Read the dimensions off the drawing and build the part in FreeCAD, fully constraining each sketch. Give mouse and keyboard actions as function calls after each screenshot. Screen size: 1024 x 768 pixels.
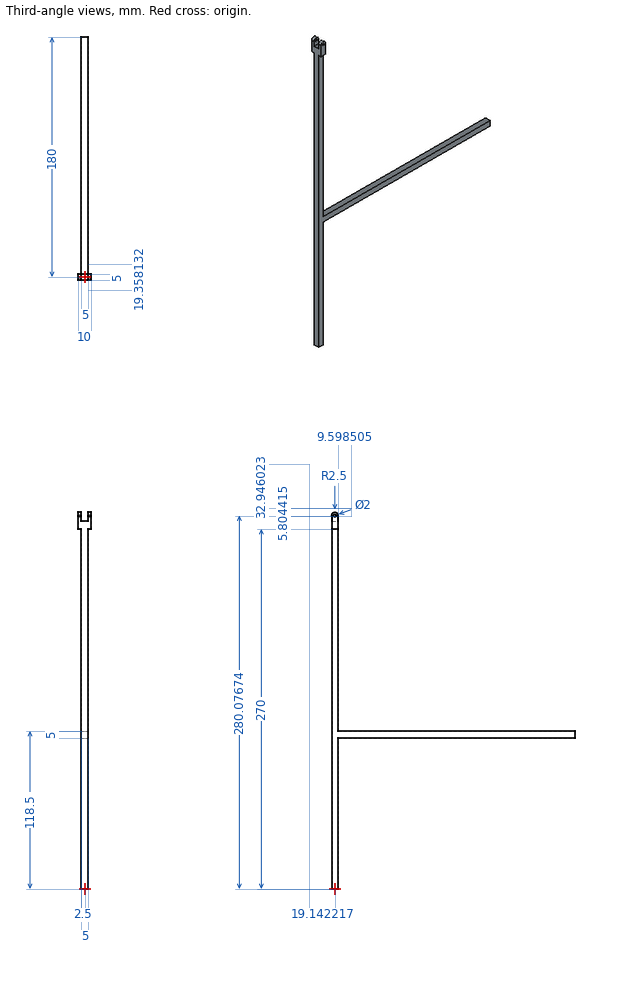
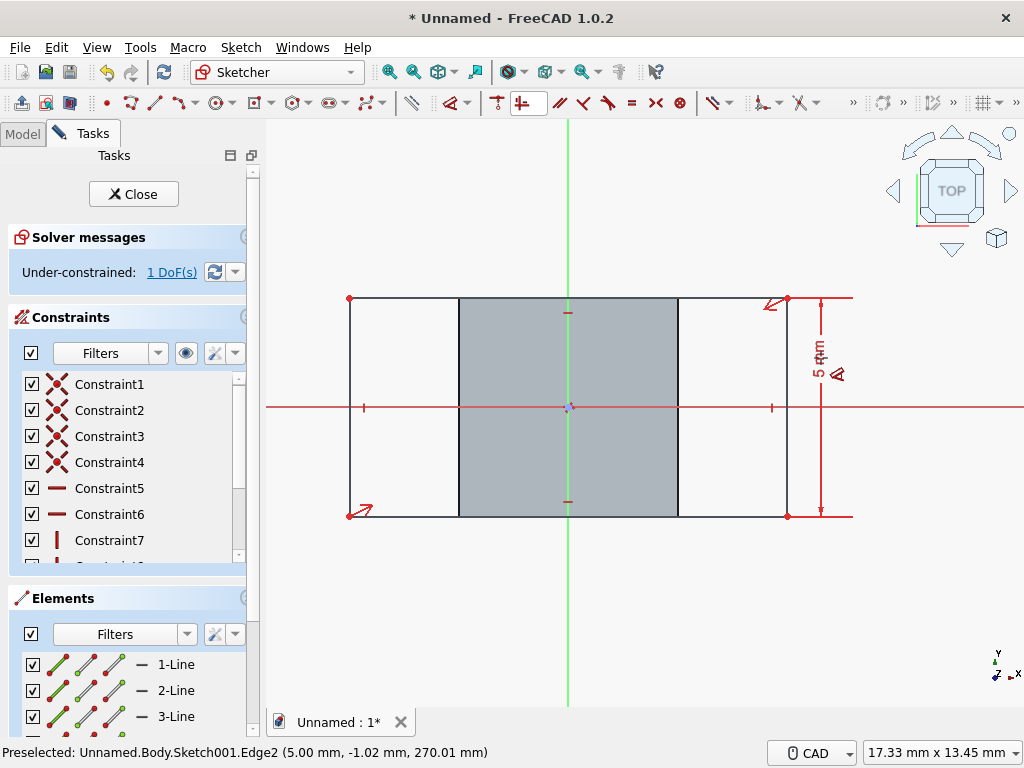
click(481, 517)
click(468, 551)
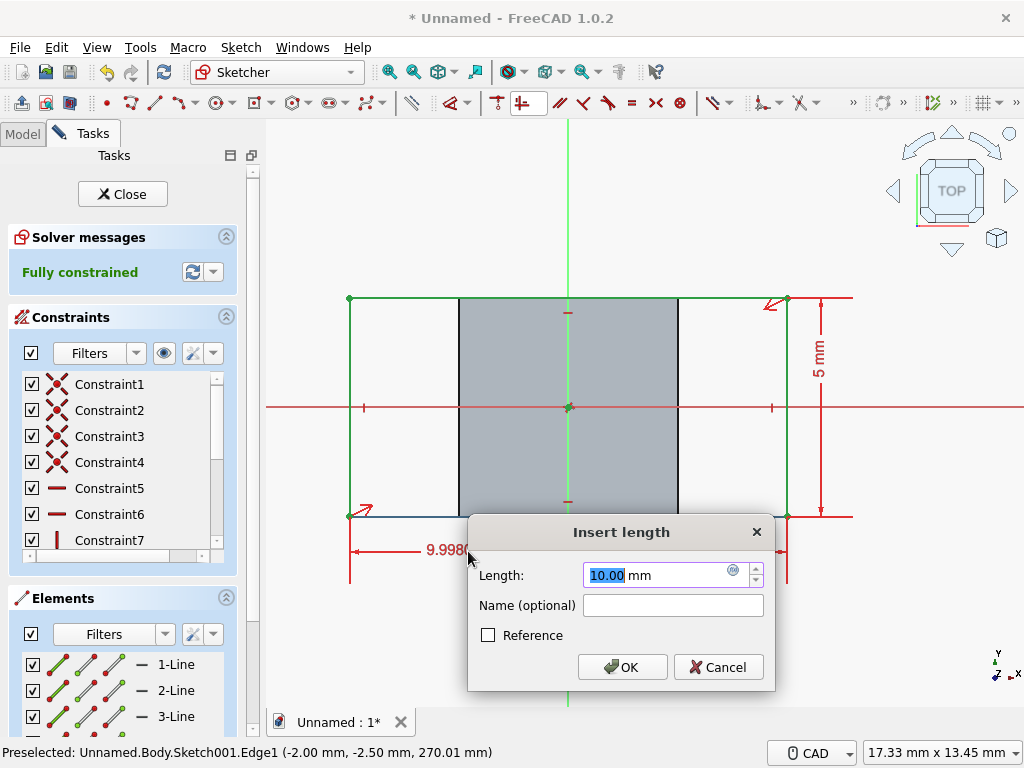
text(10)
key(Return)
key(Escape)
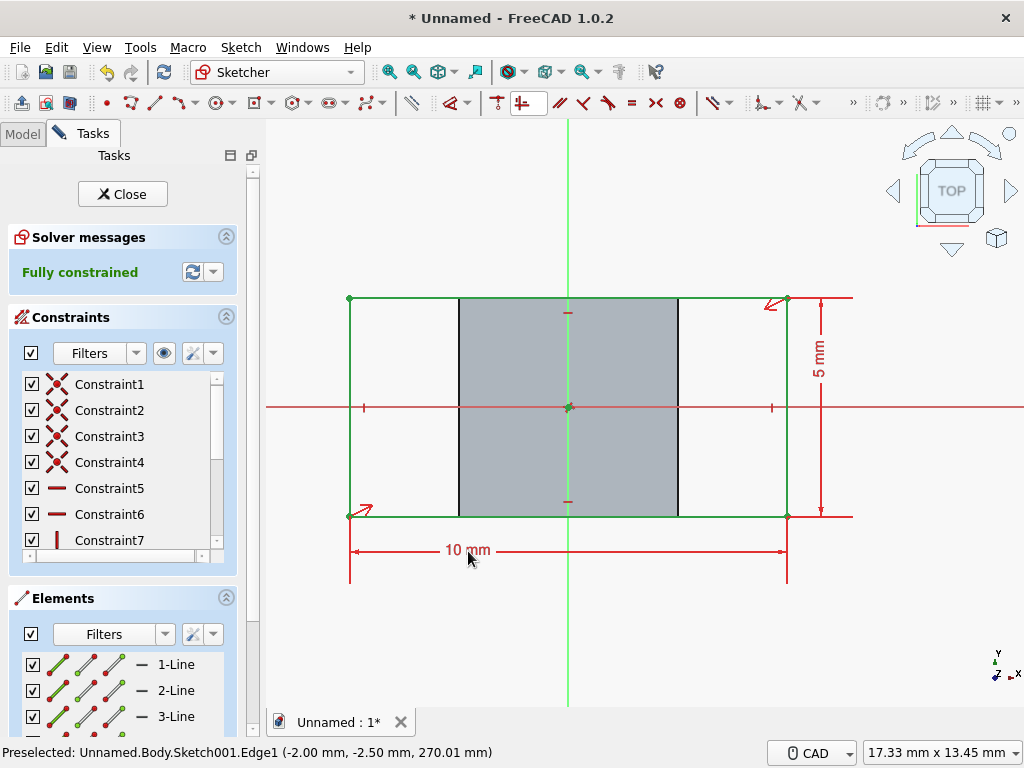
click(123, 194)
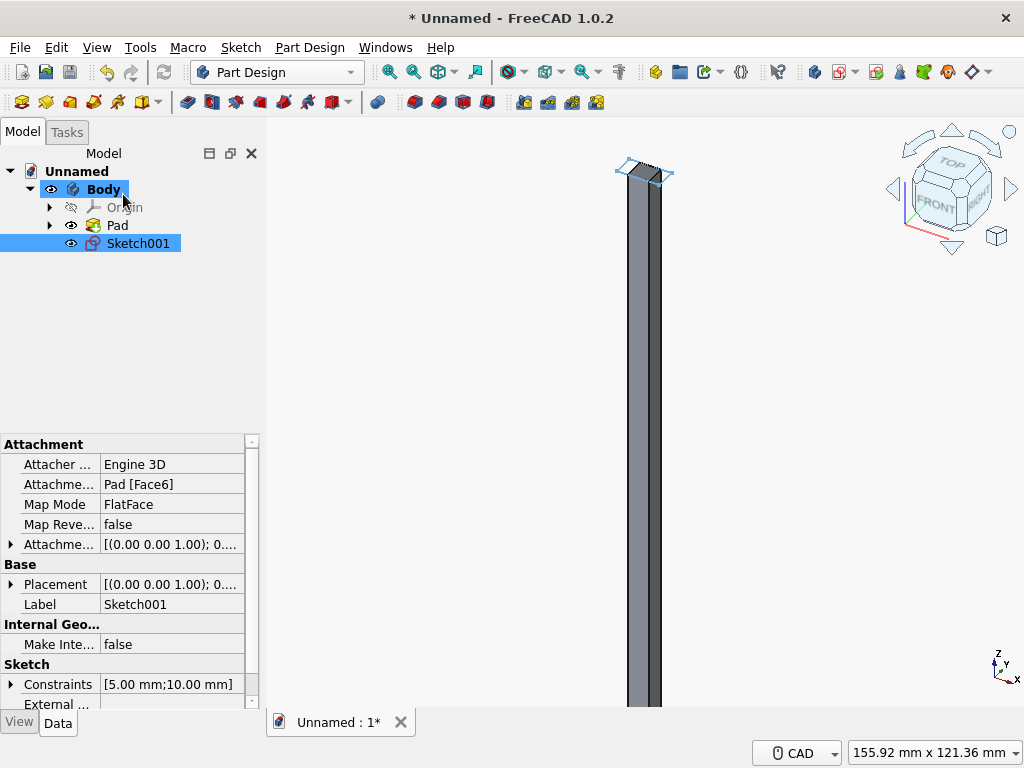
click(22, 102)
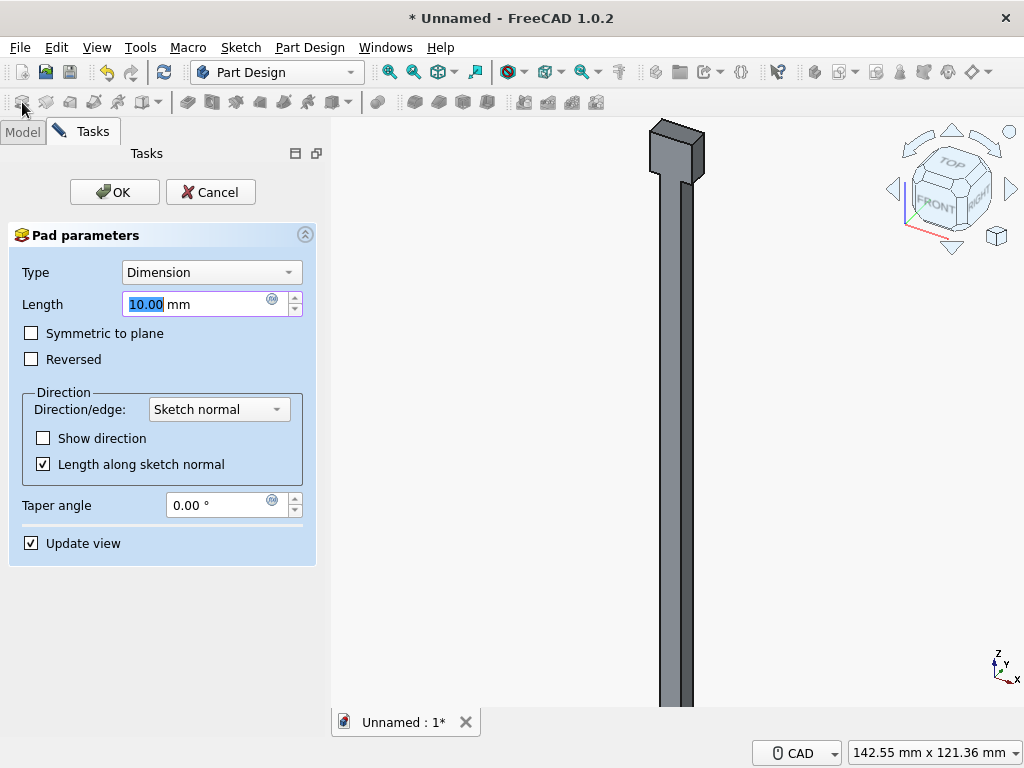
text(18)
key(Tab)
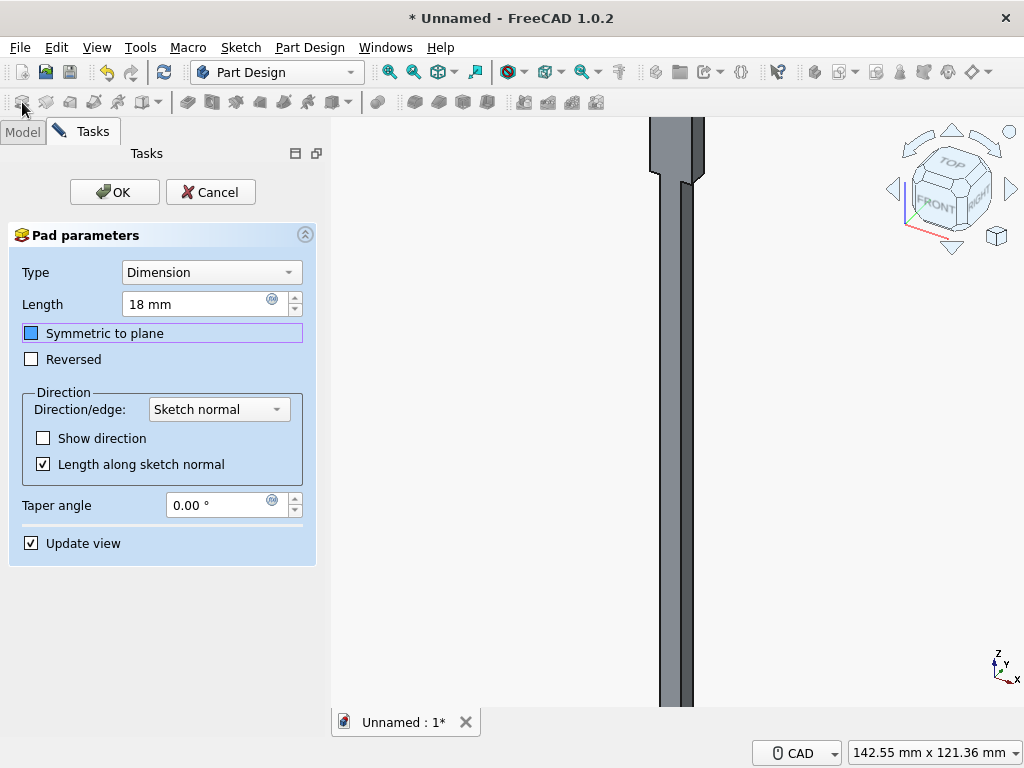
click(115, 192)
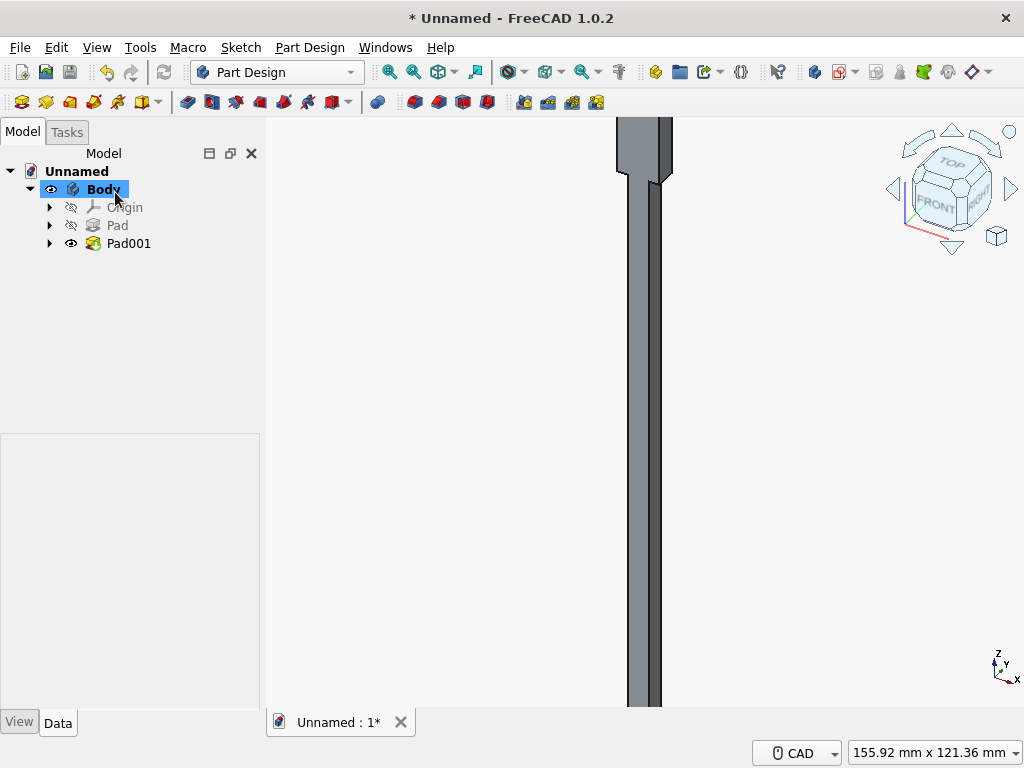
click(390, 72)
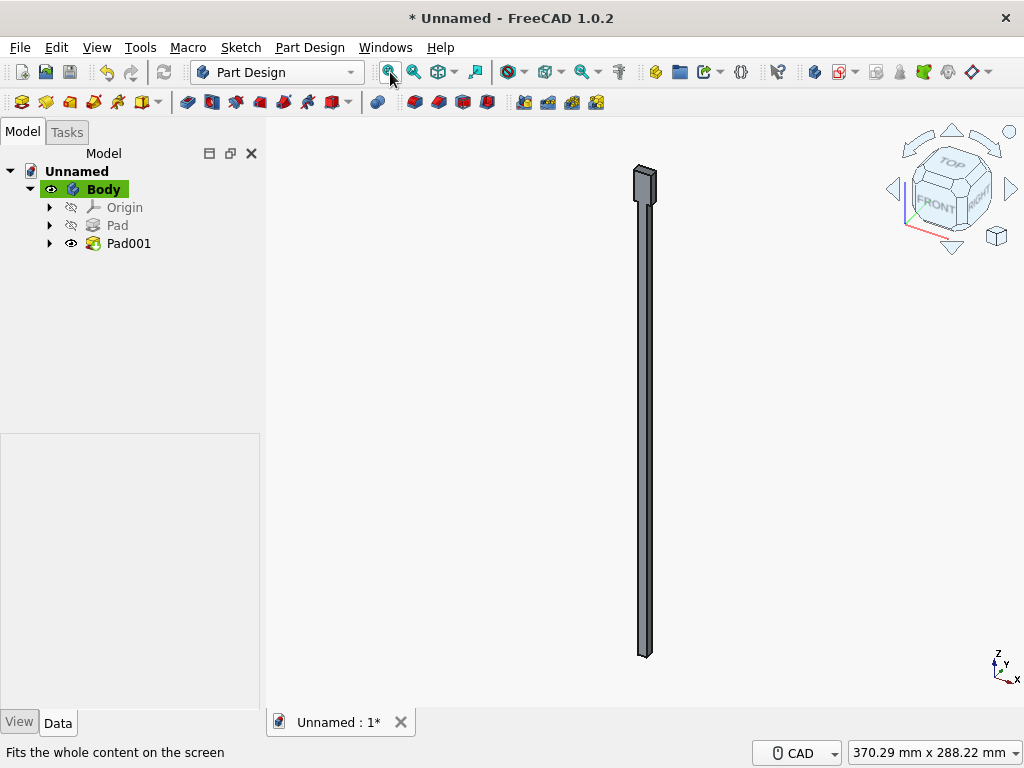
scroll(648, 170, up, 5)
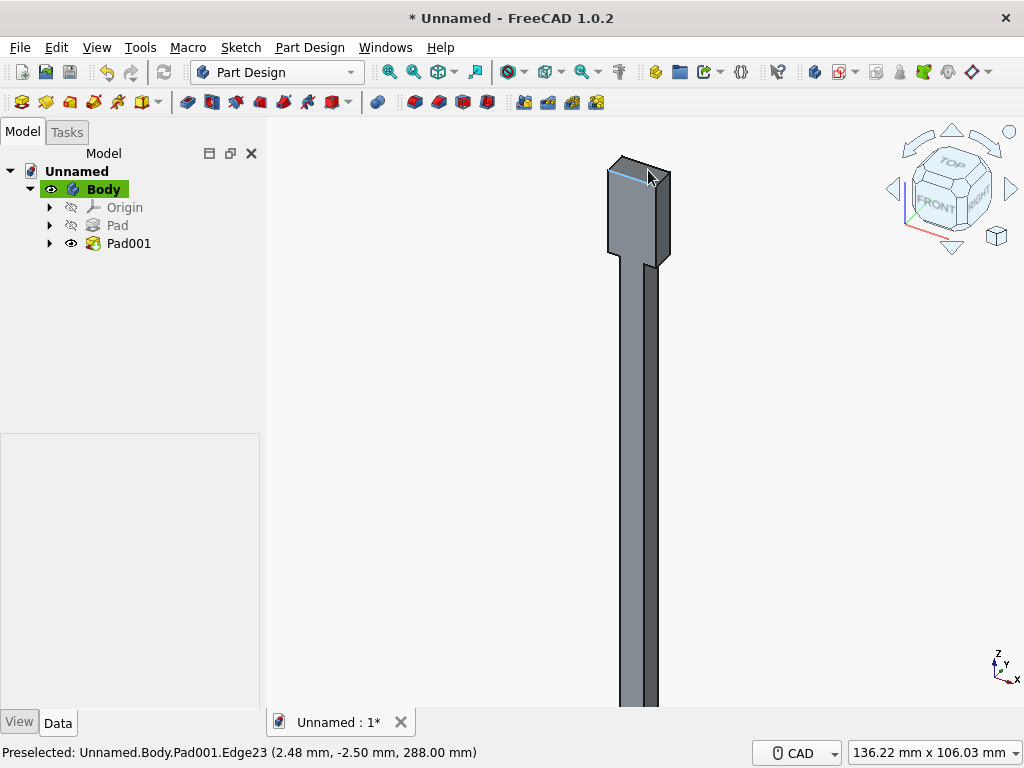
click(639, 170)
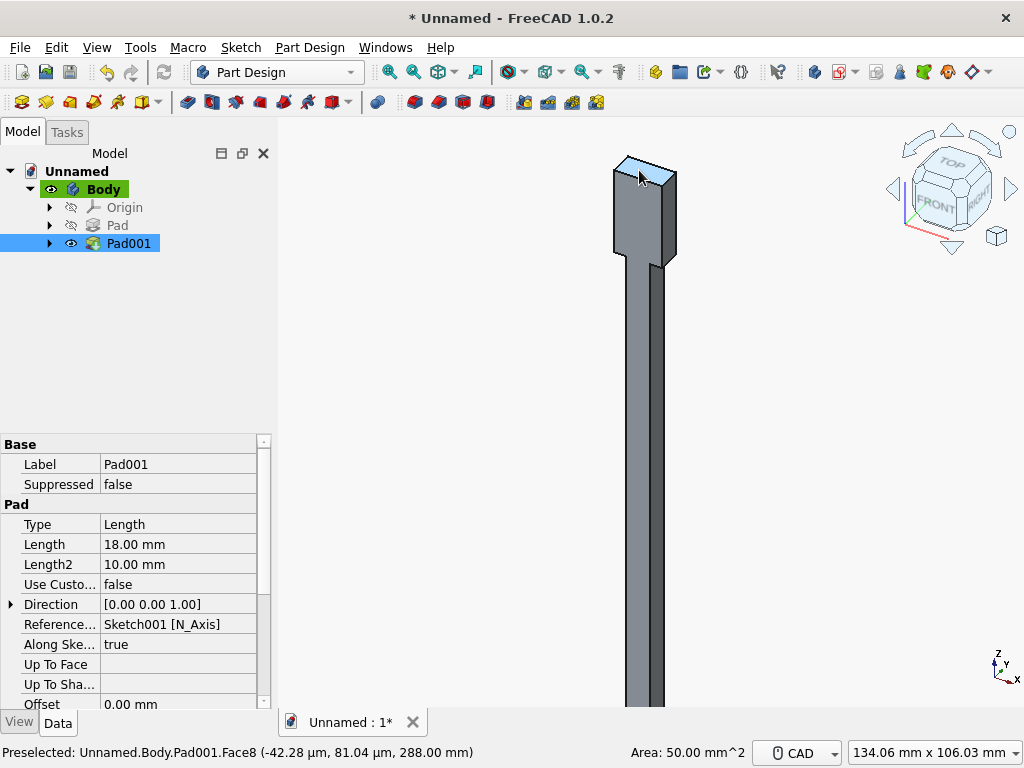
click(840, 72)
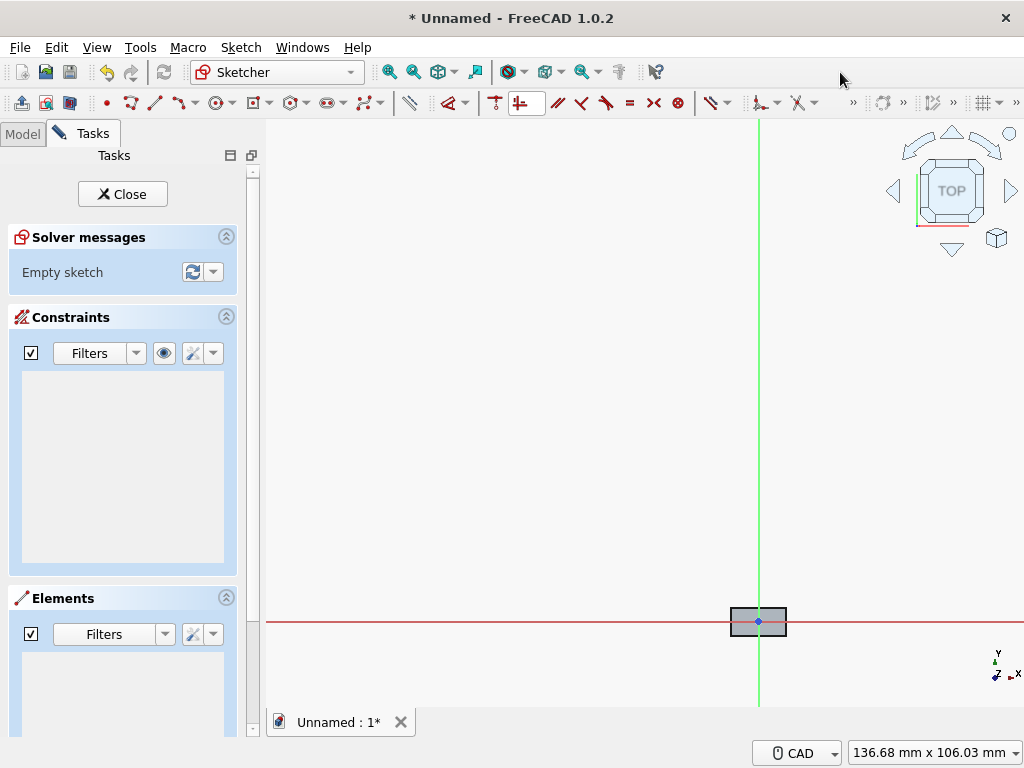
scroll(576, 413, down, 5)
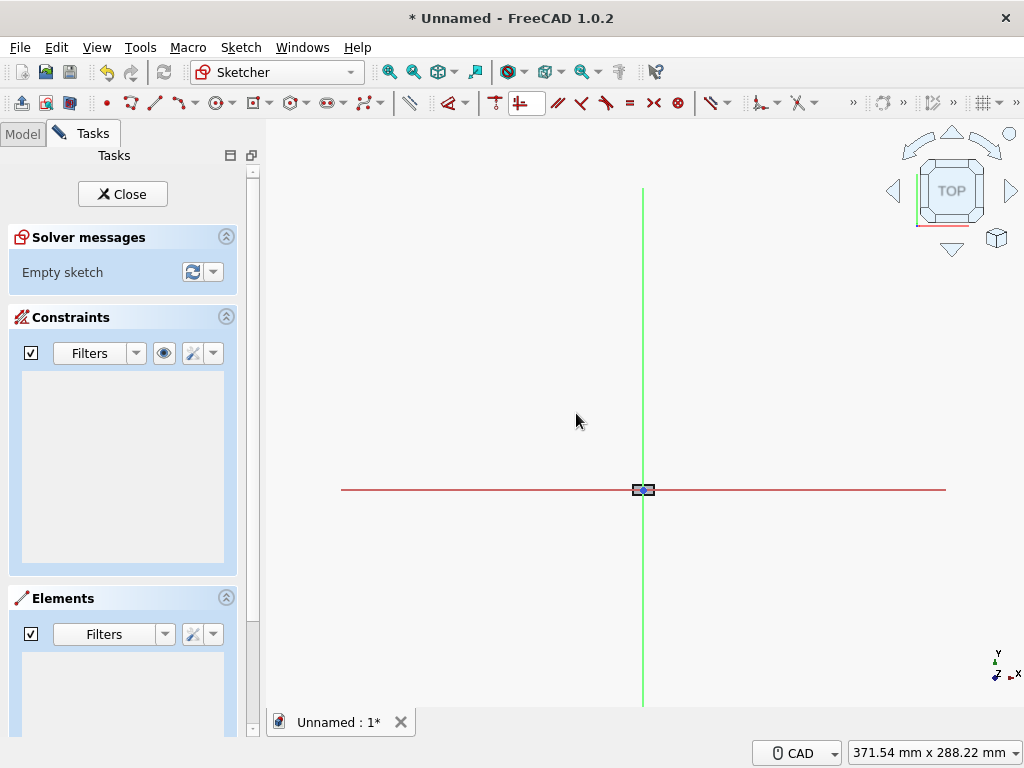
scroll(652, 500, up, 11)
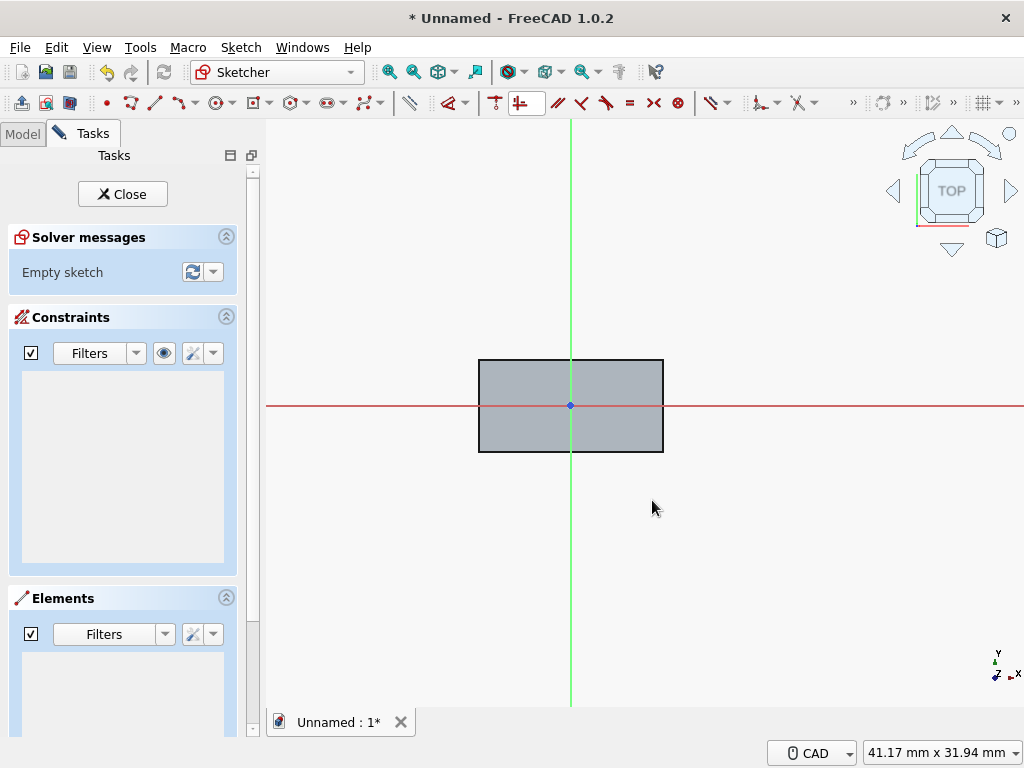
click(254, 104)